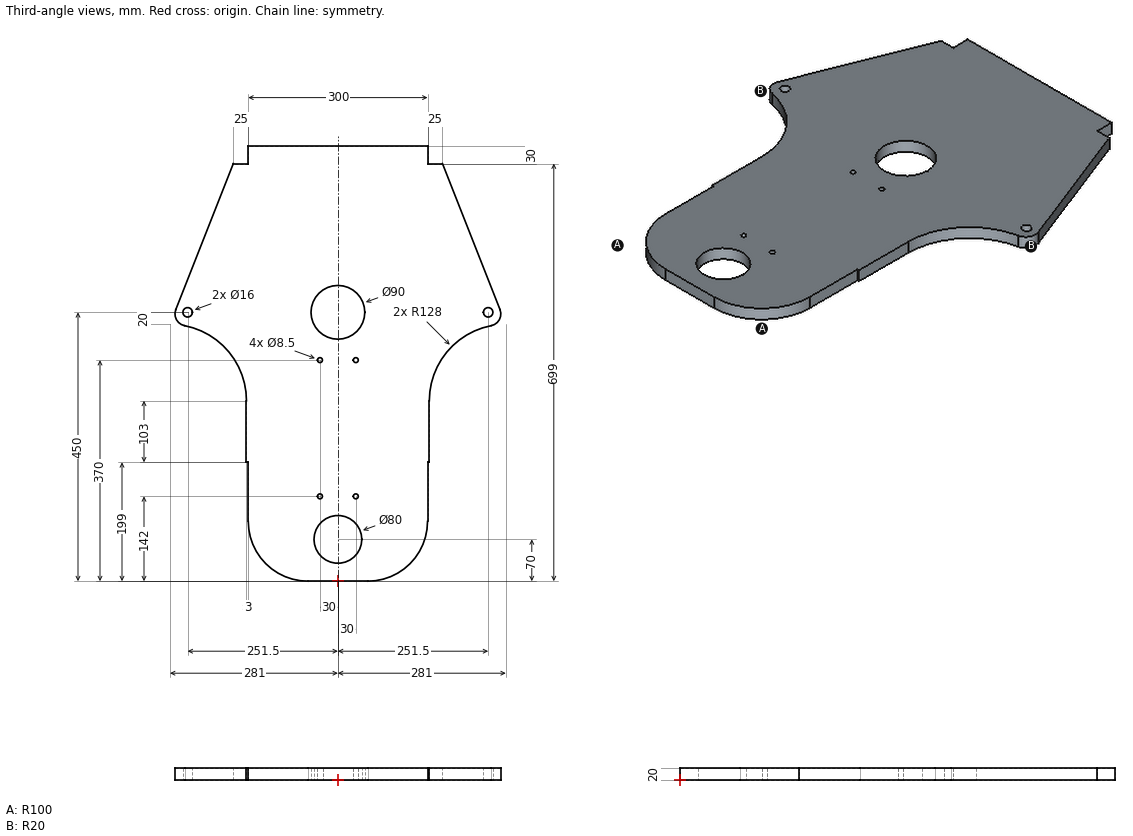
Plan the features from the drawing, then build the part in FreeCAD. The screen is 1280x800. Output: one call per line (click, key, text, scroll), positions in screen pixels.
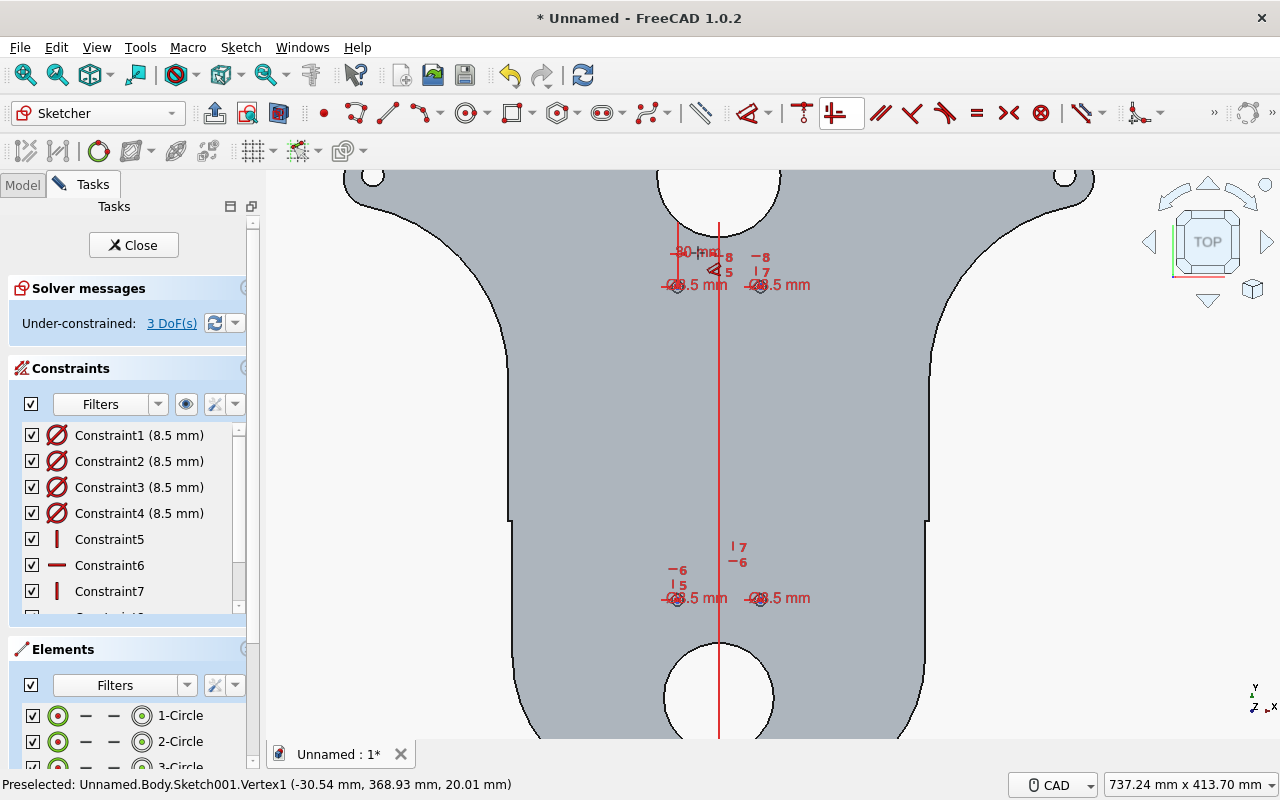
click(760, 600)
click(740, 566)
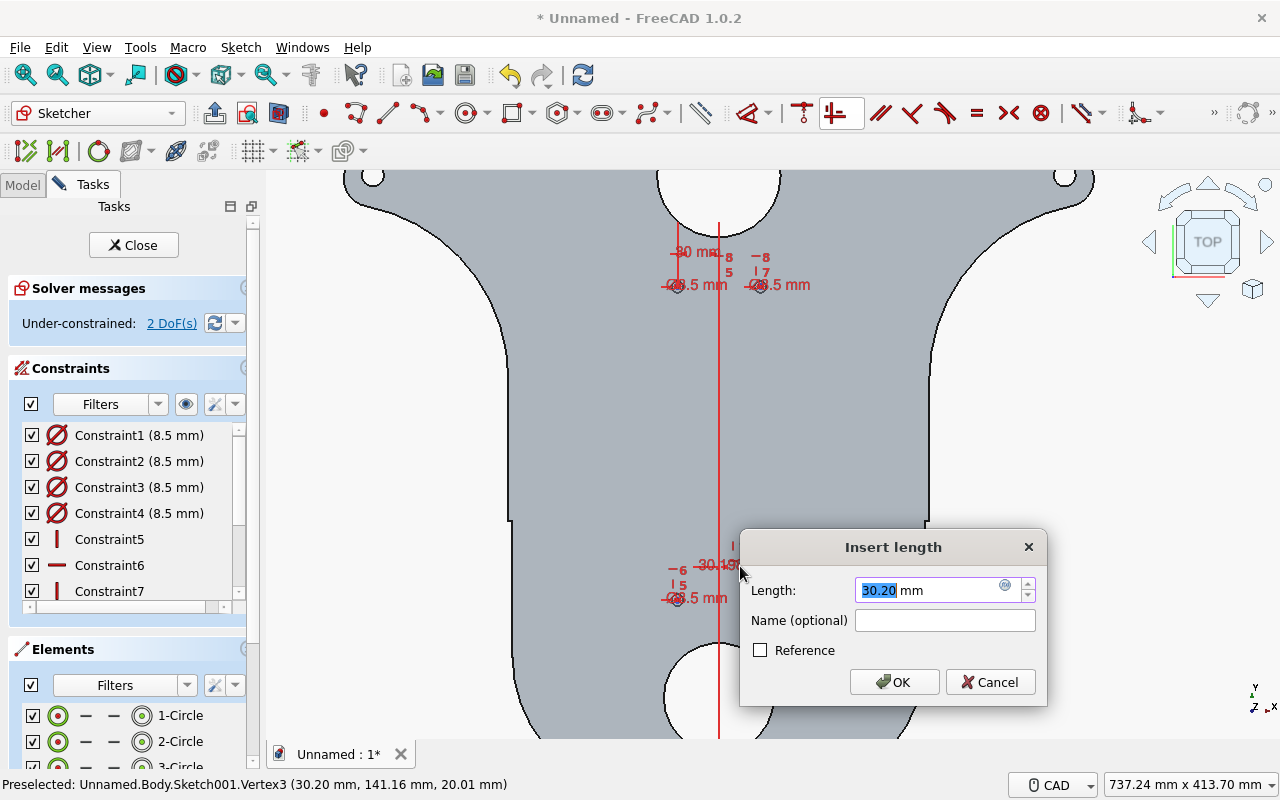
text(30)
key(Return)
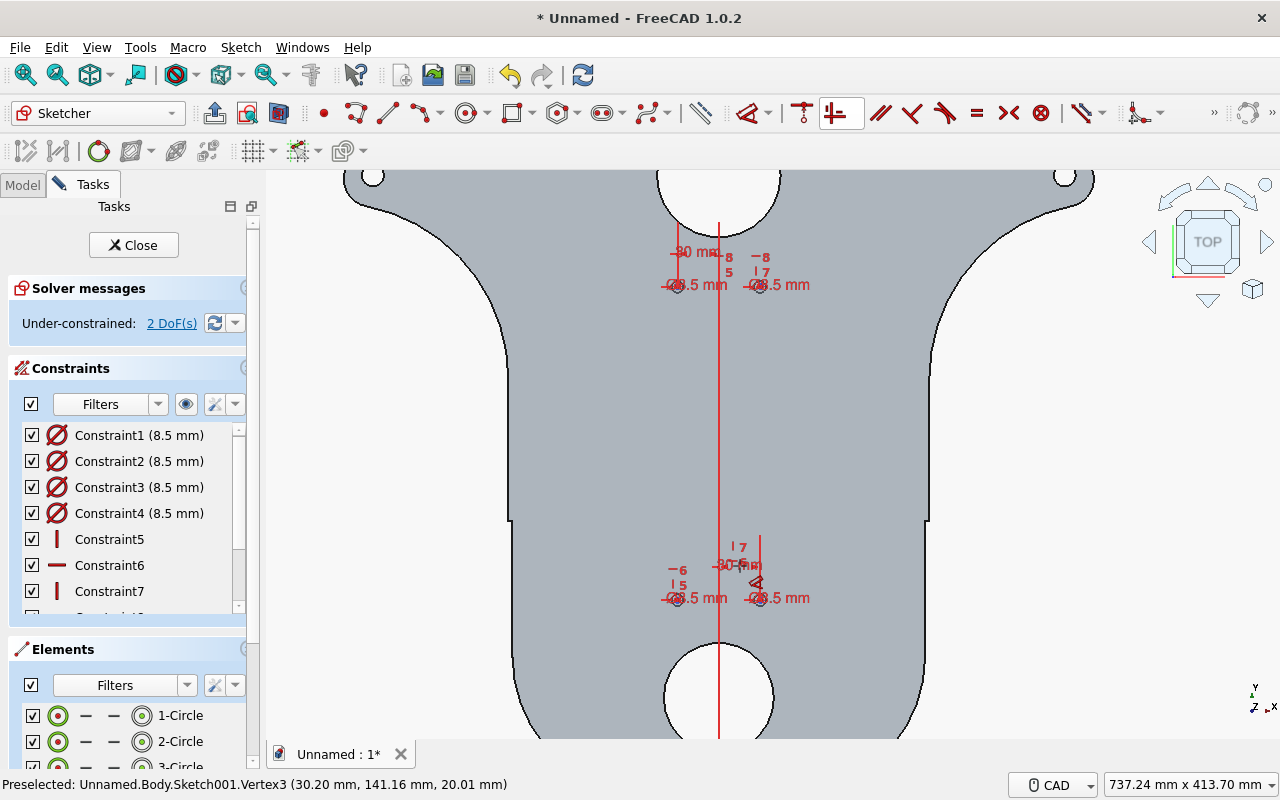
click(678, 287)
click(644, 499)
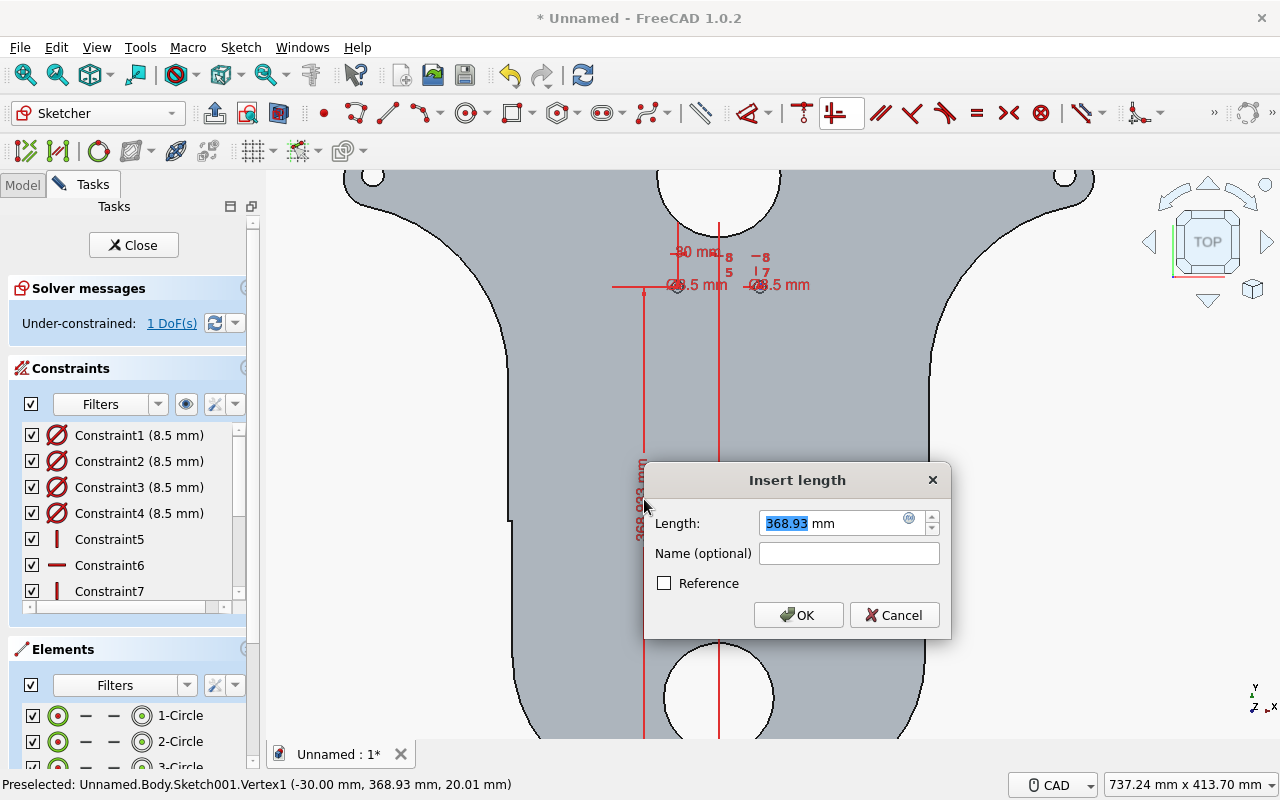
text(370)
key(Return)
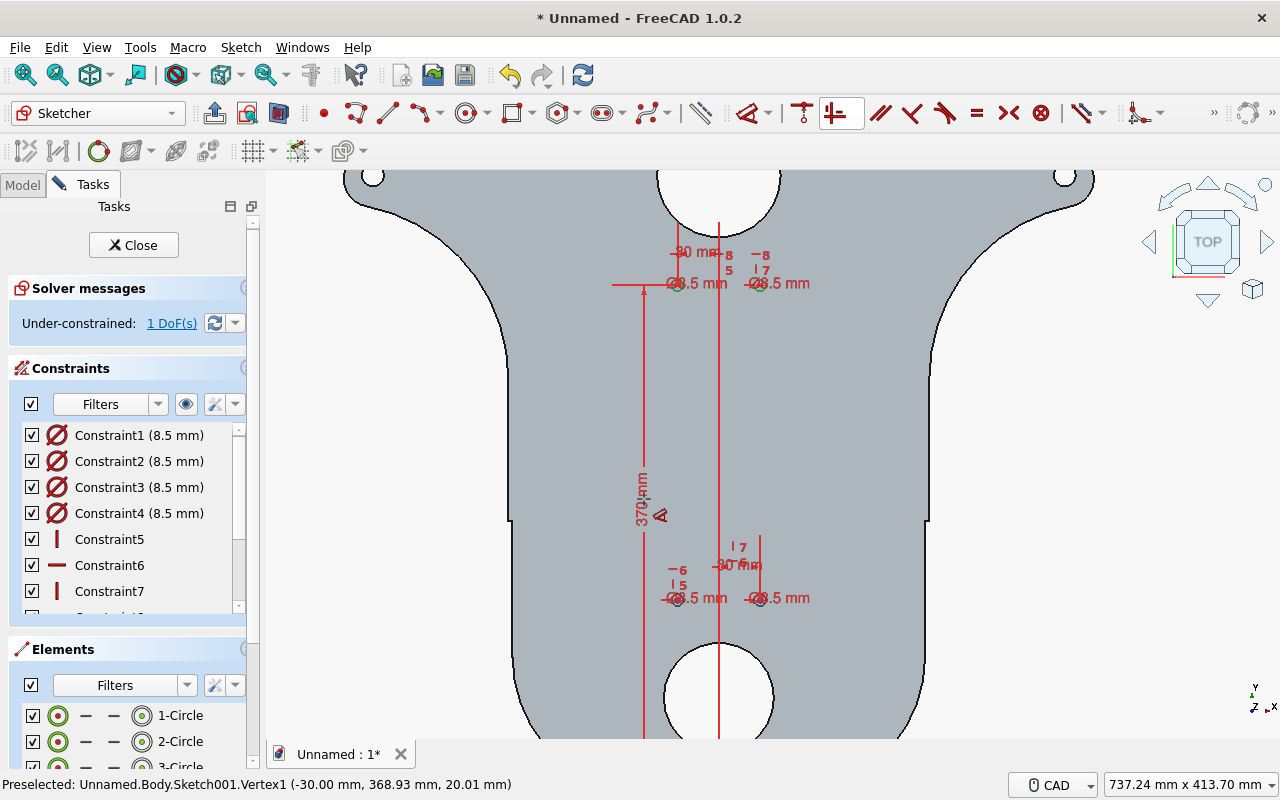
click(678, 600)
click(644, 656)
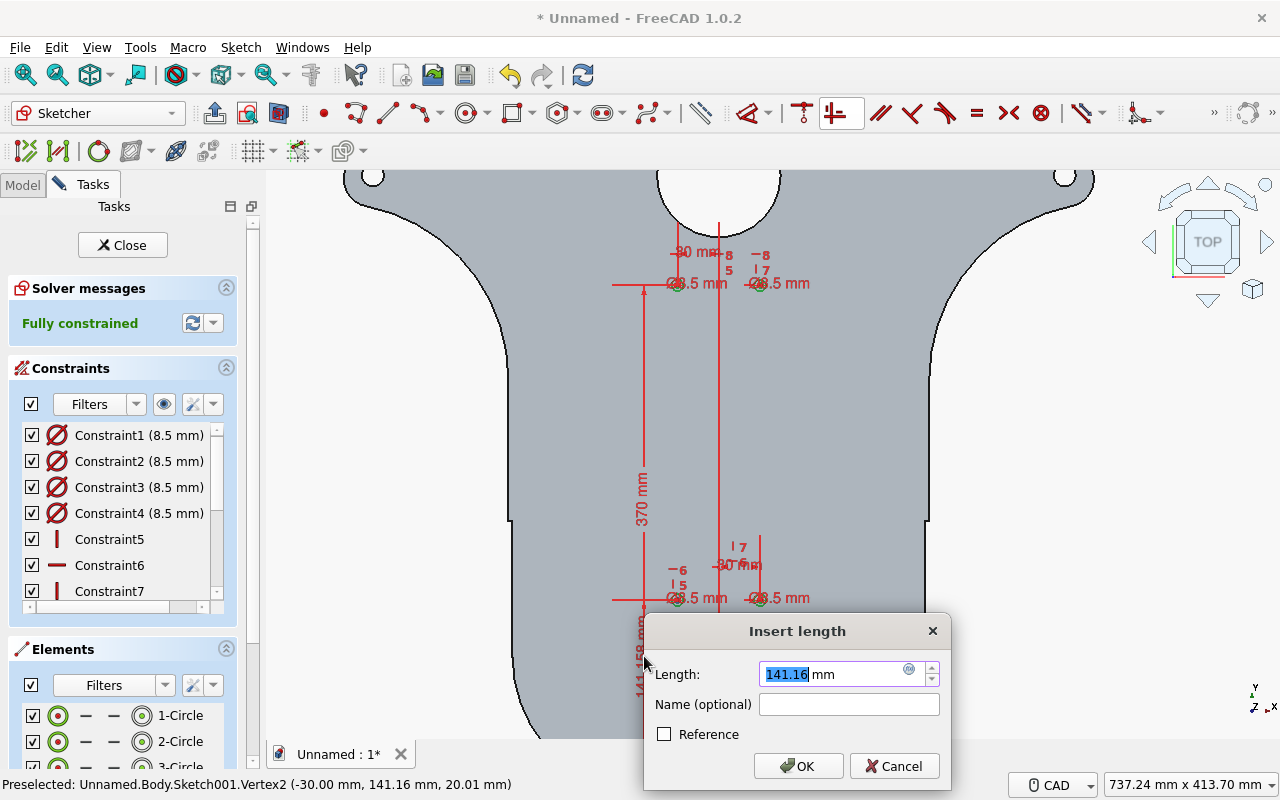
text(142)
key(Return)
key(Escape)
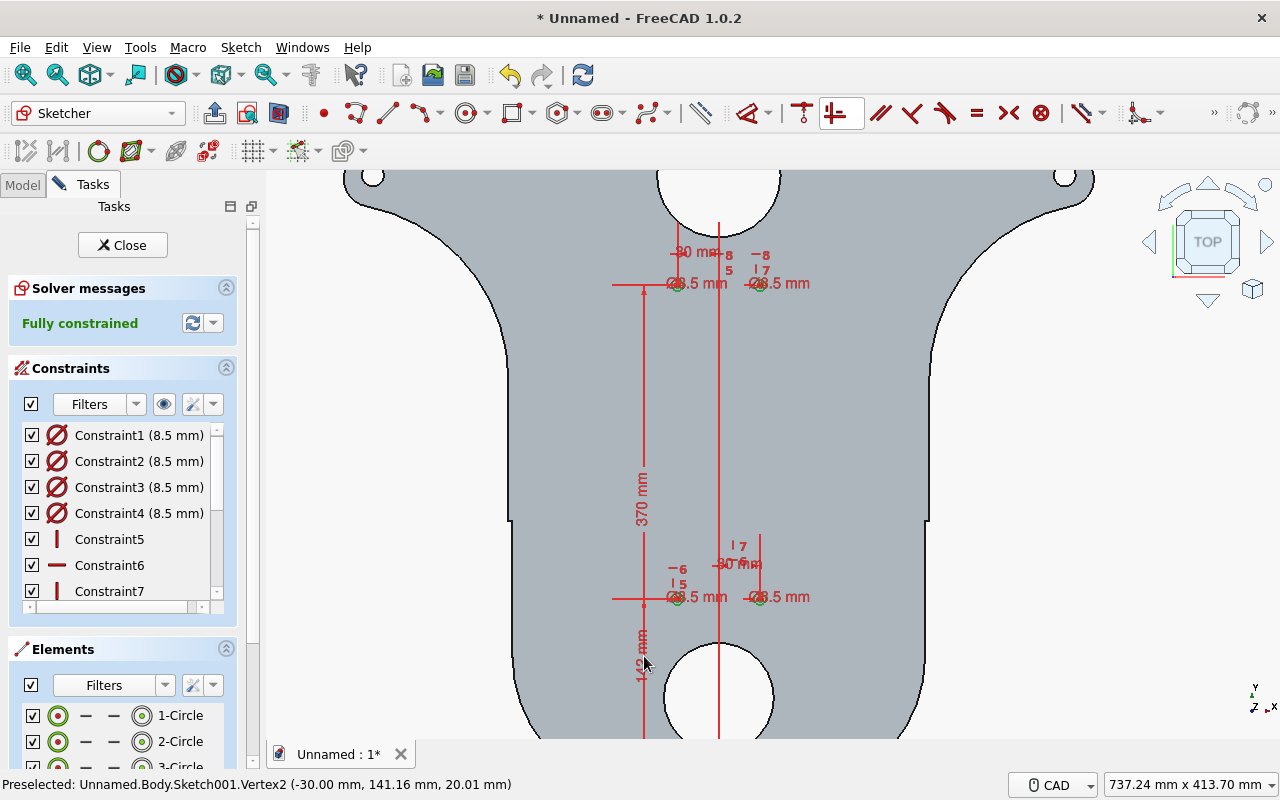
click(123, 245)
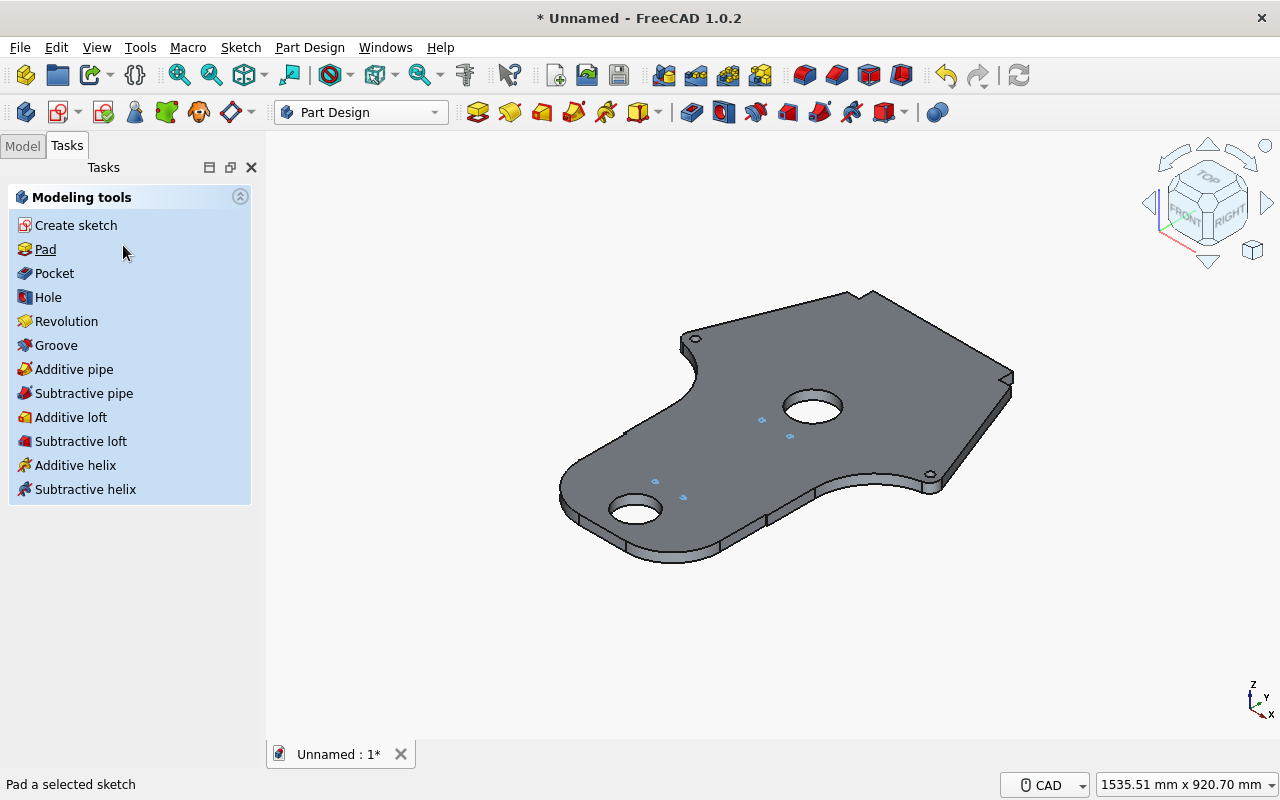
click(692, 112)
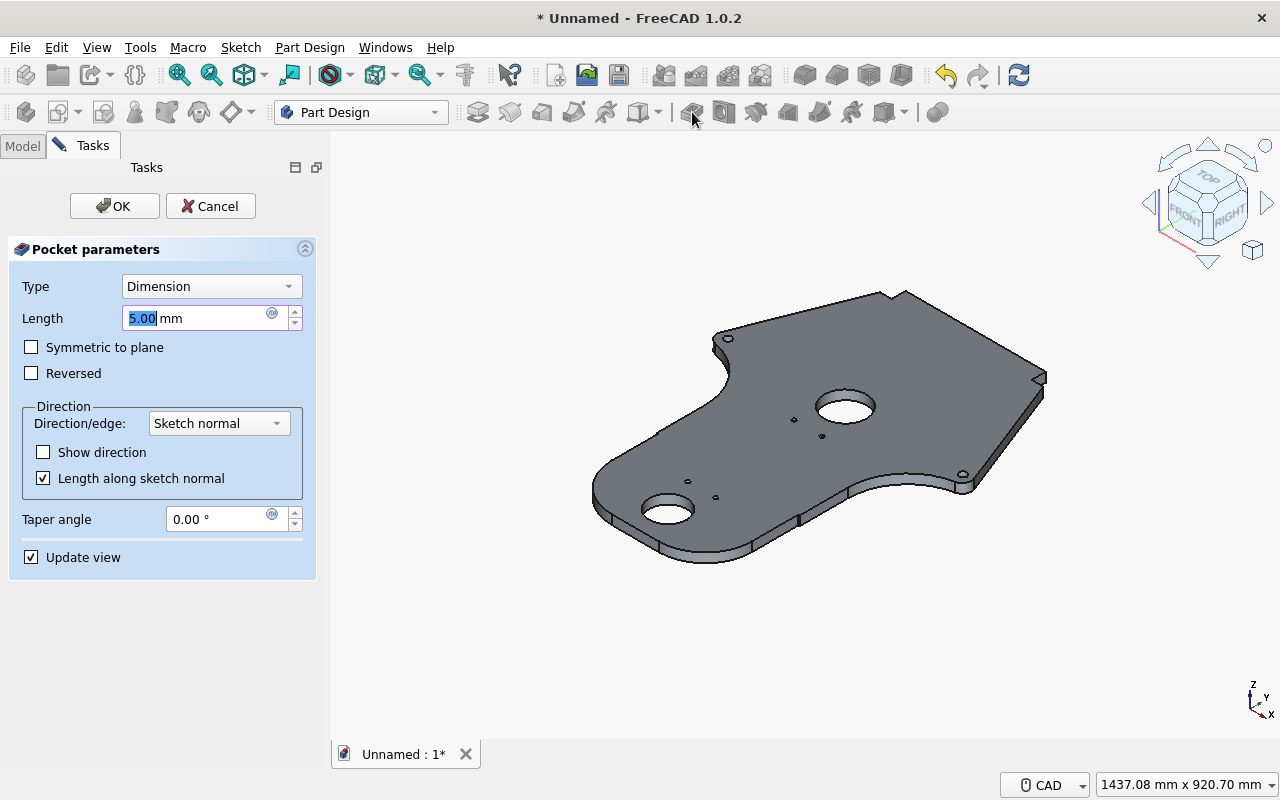
click(212, 286)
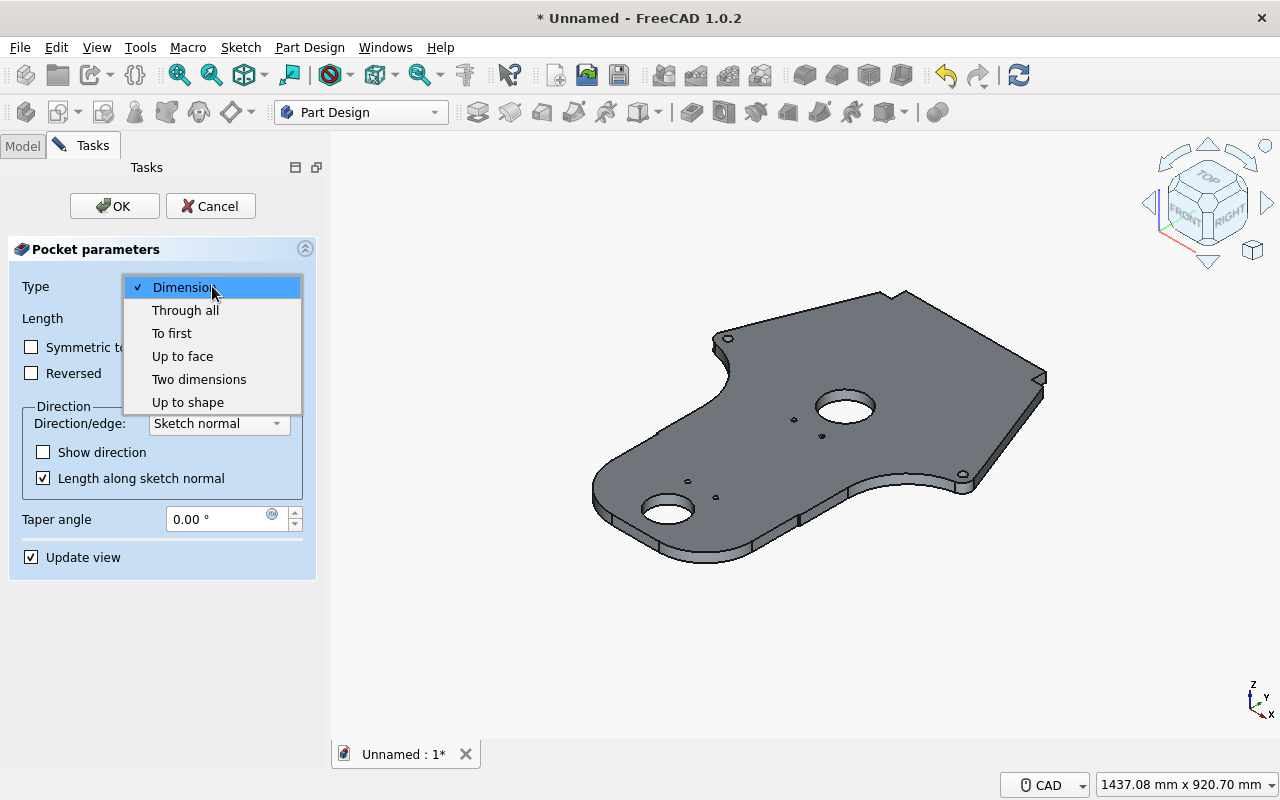
click(212, 310)